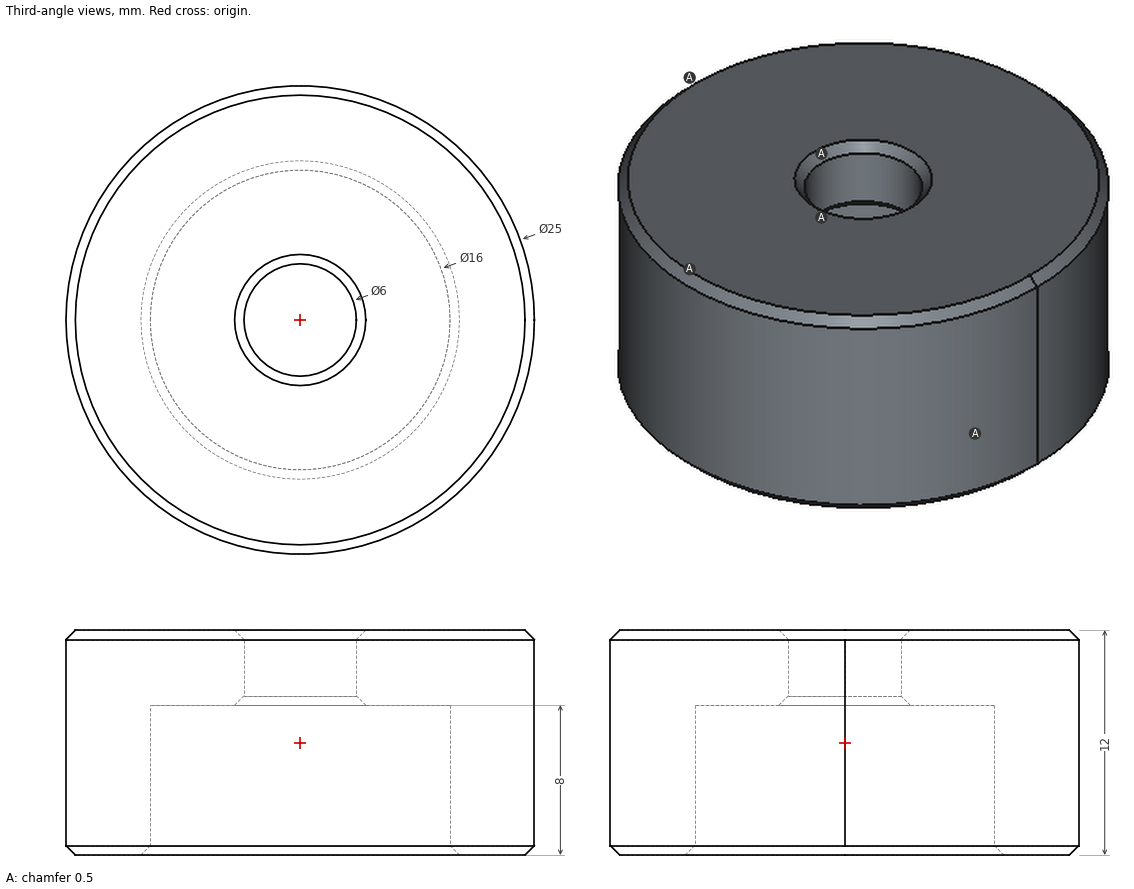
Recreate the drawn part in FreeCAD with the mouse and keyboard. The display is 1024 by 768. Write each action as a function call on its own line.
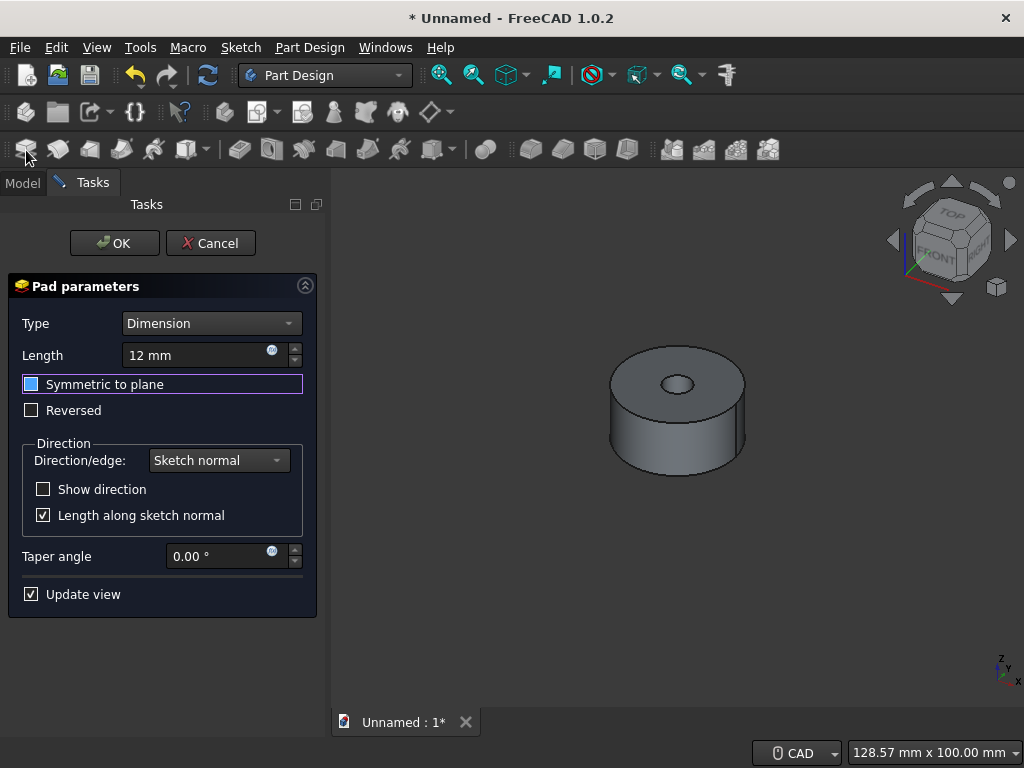
click(30, 384)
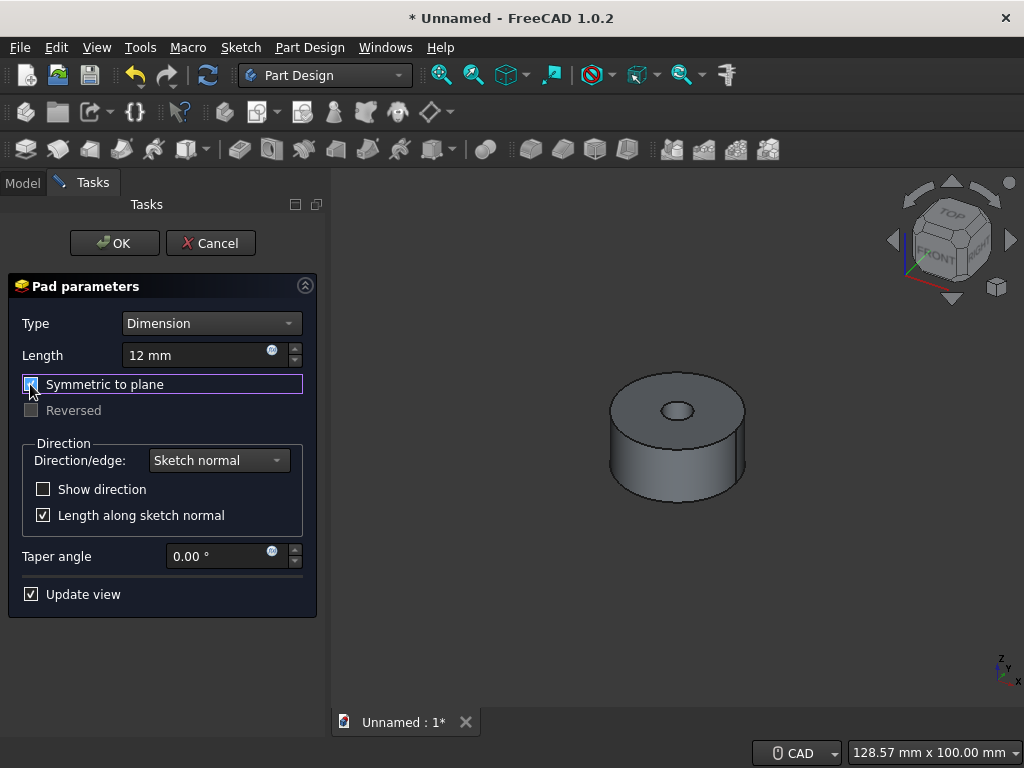
click(115, 243)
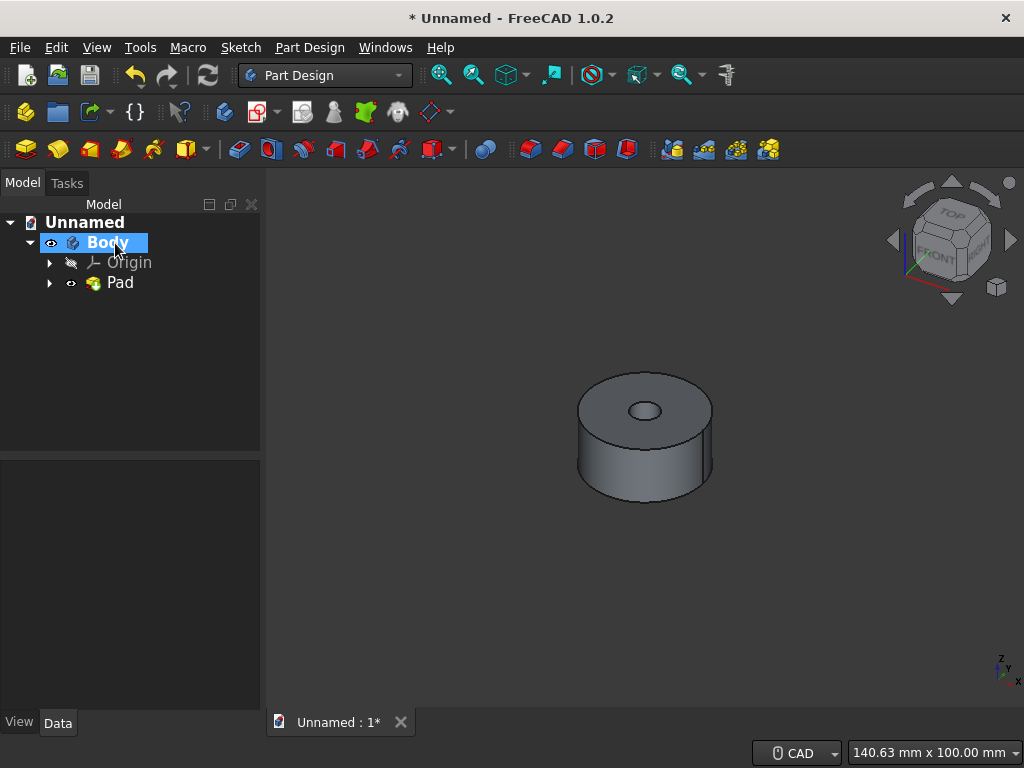
key(v)
key(f)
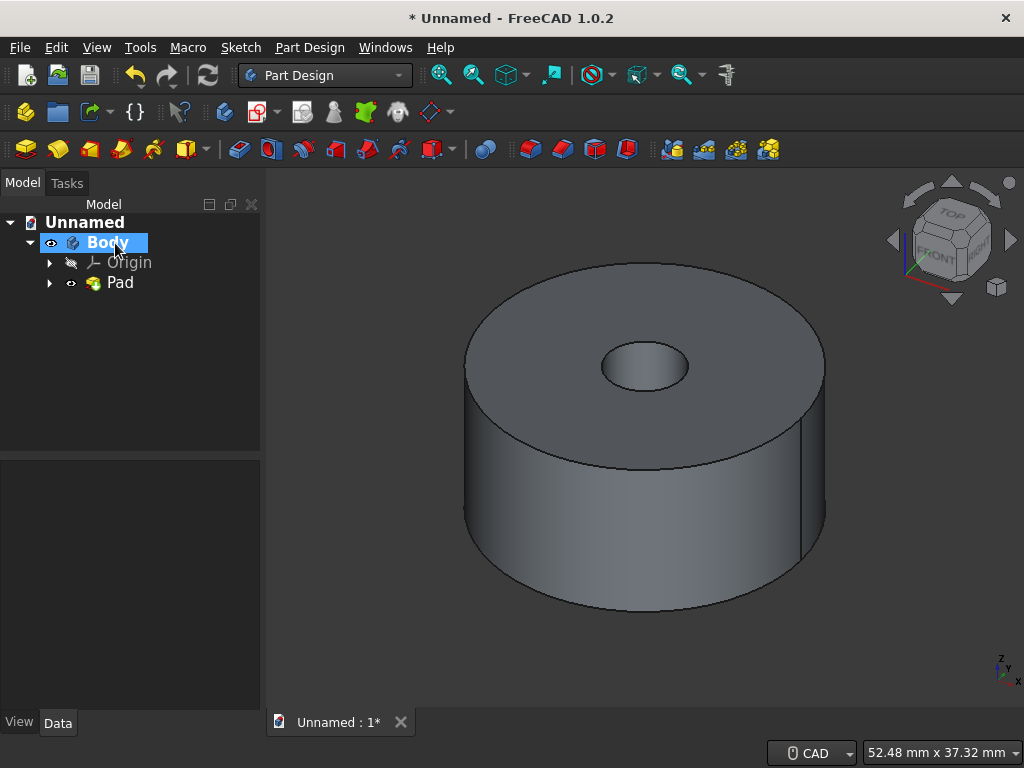
key(5)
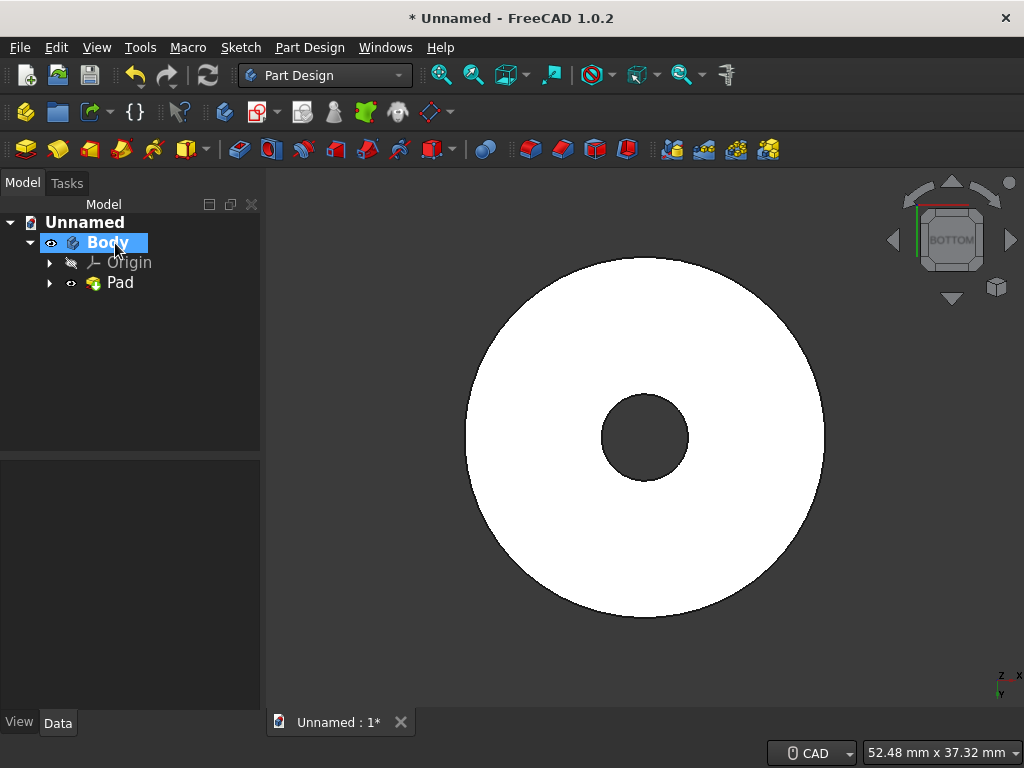
click(748, 385)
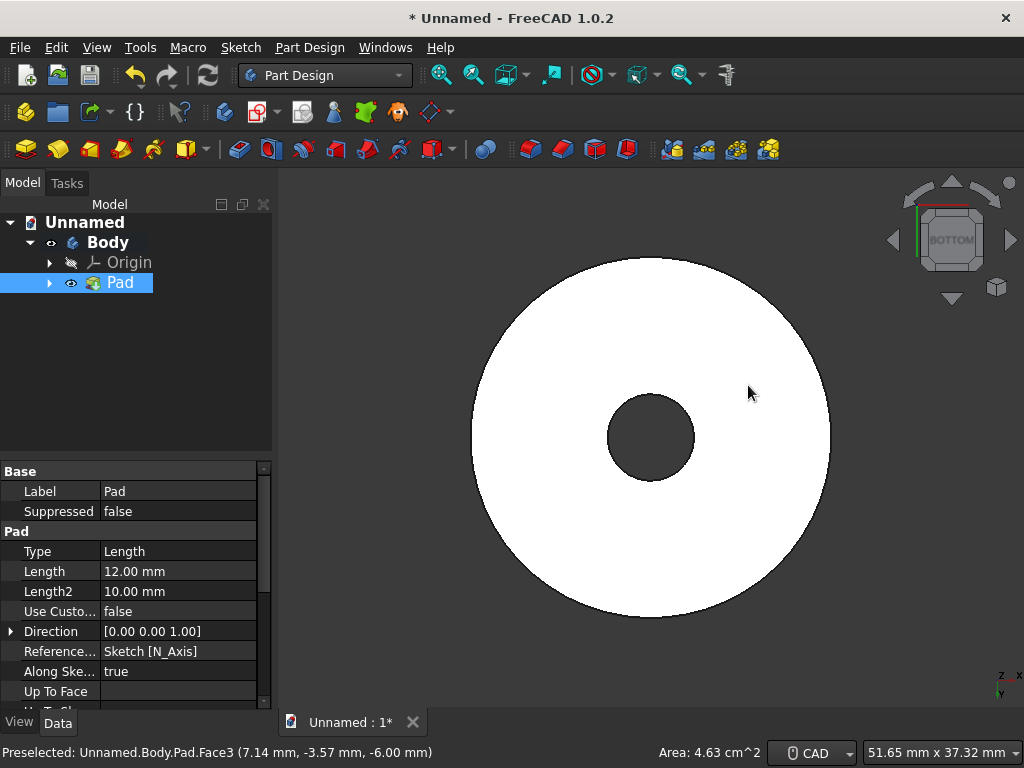
click(258, 112)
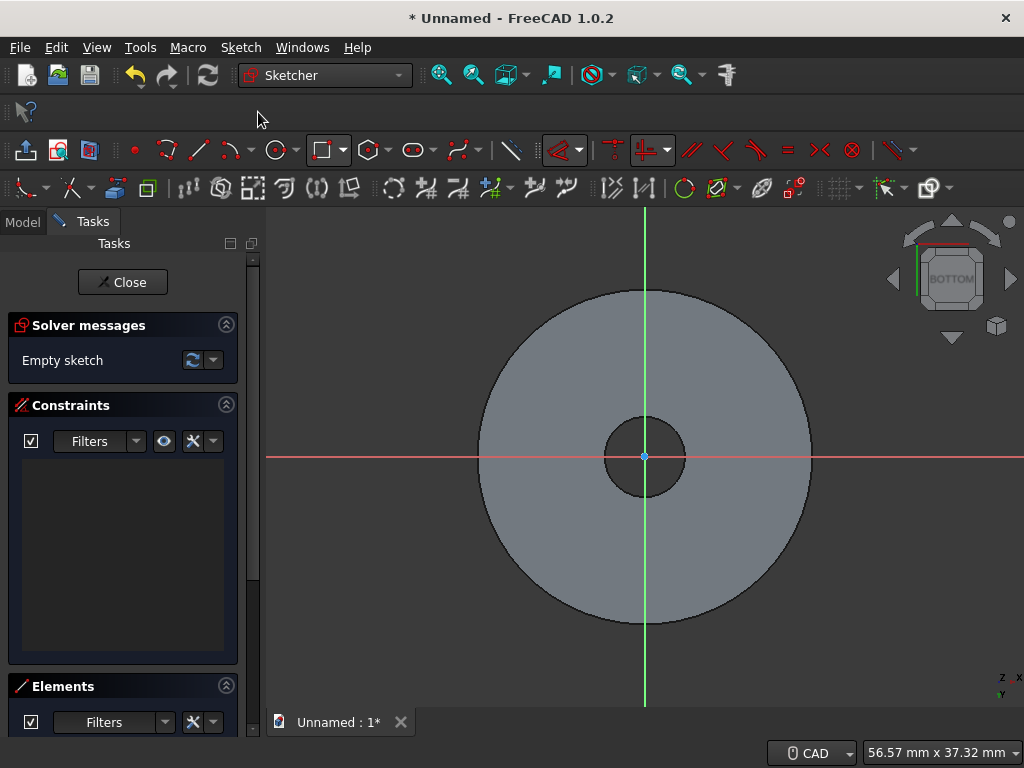
scroll(784, 457, up, 2)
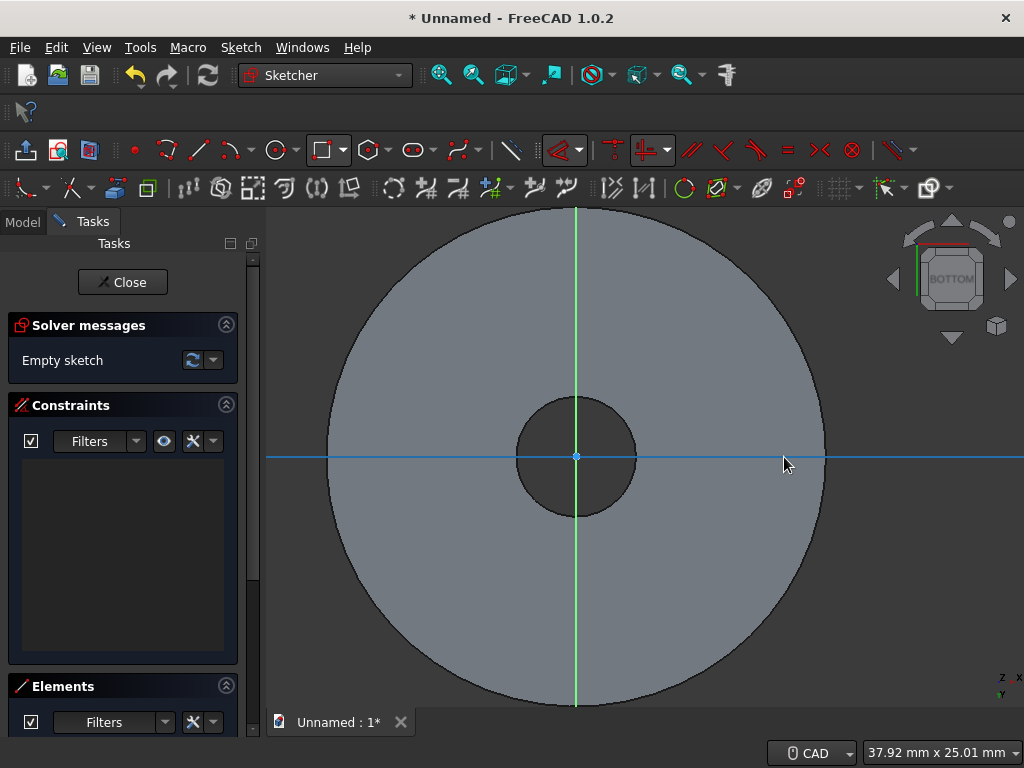
click(276, 150)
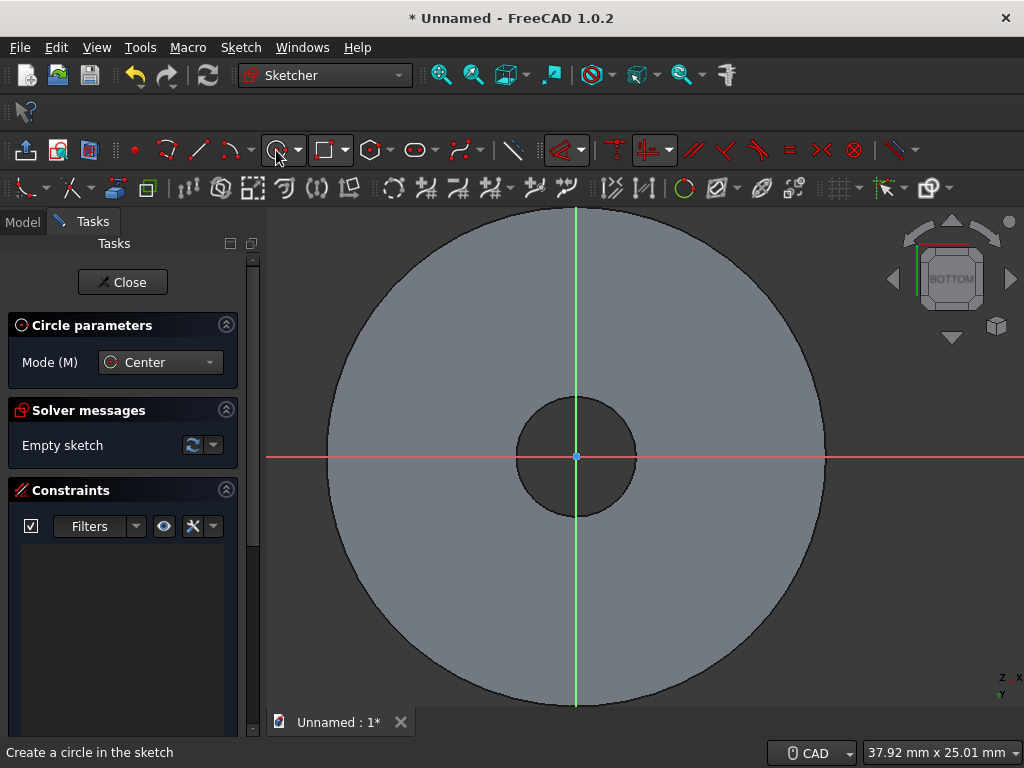
click(576, 457)
move(689, 344)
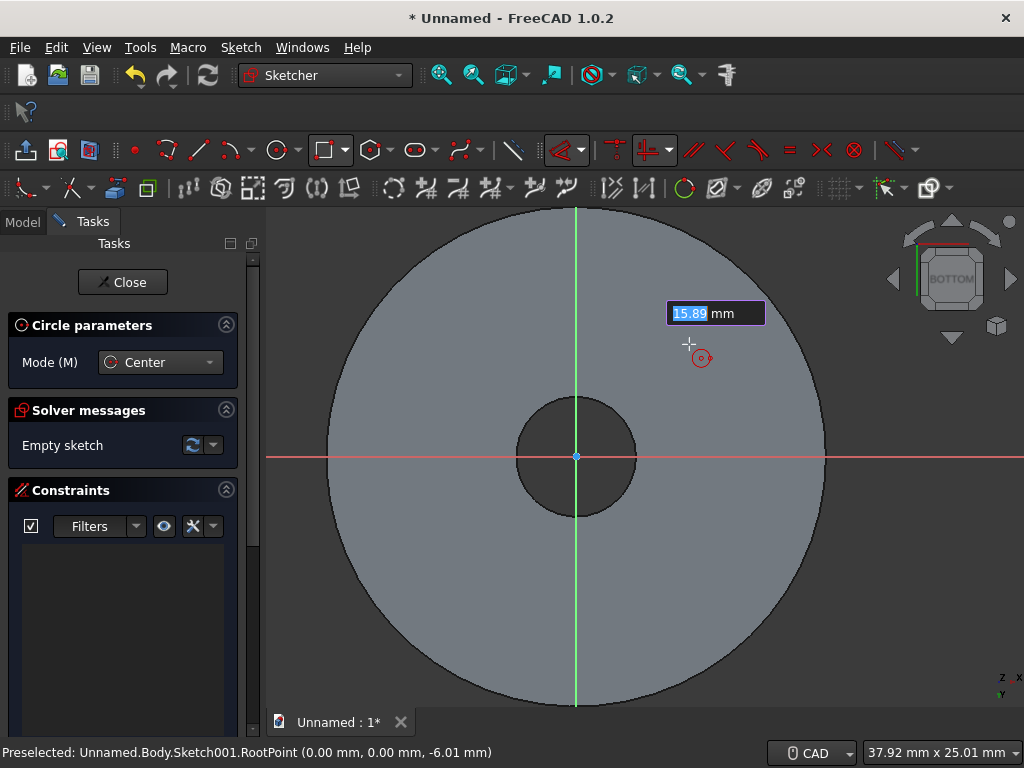
text(16)
key(Return)
key(Escape)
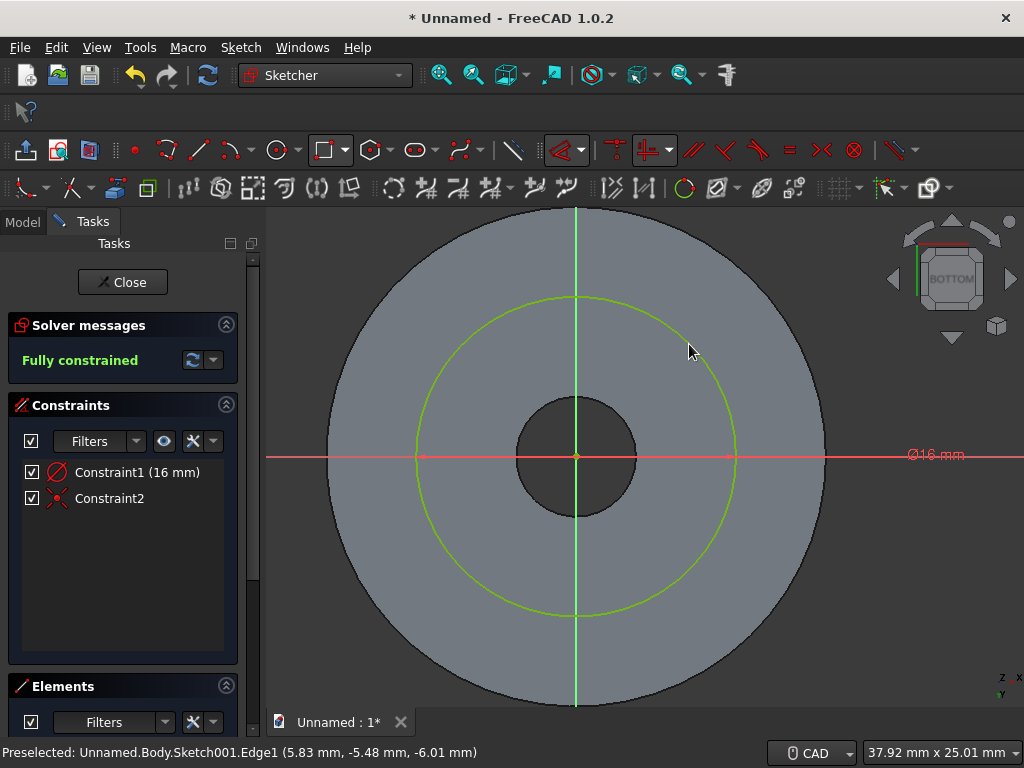
click(123, 282)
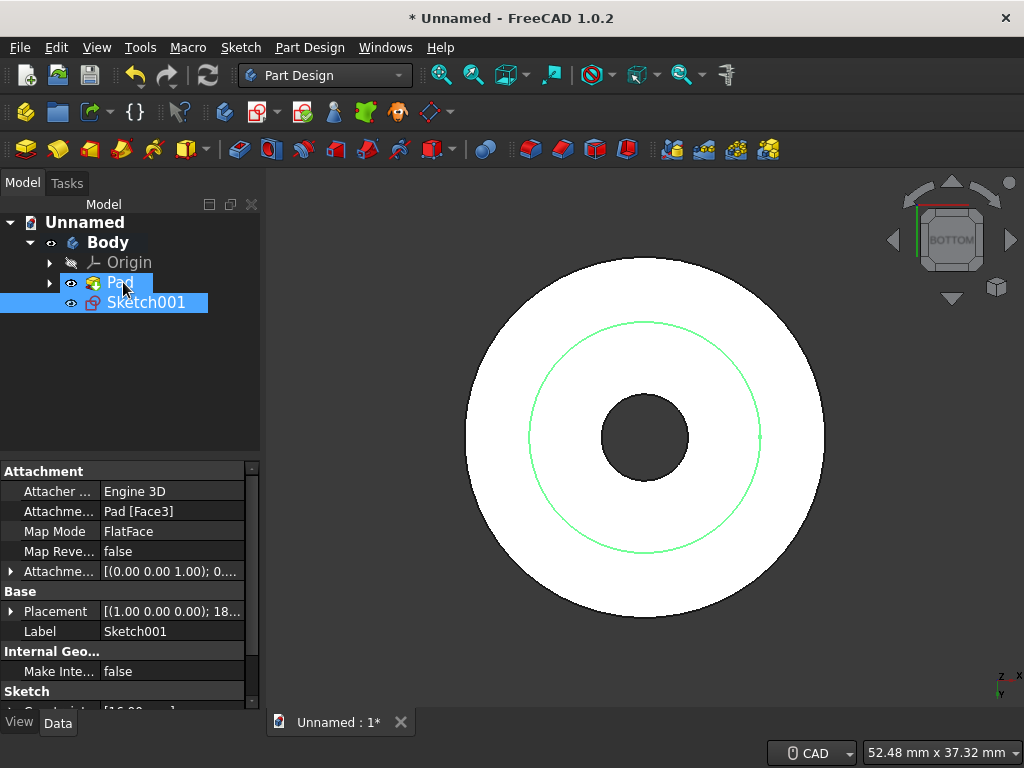
click(240, 150)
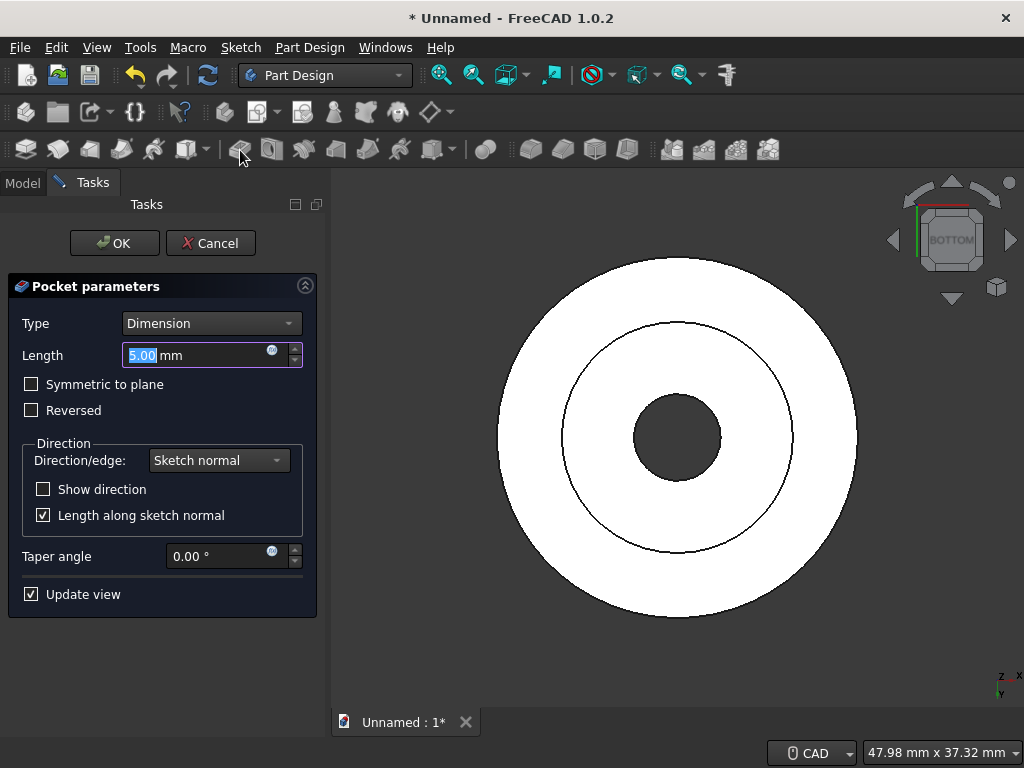
text(8)
key(Tab)